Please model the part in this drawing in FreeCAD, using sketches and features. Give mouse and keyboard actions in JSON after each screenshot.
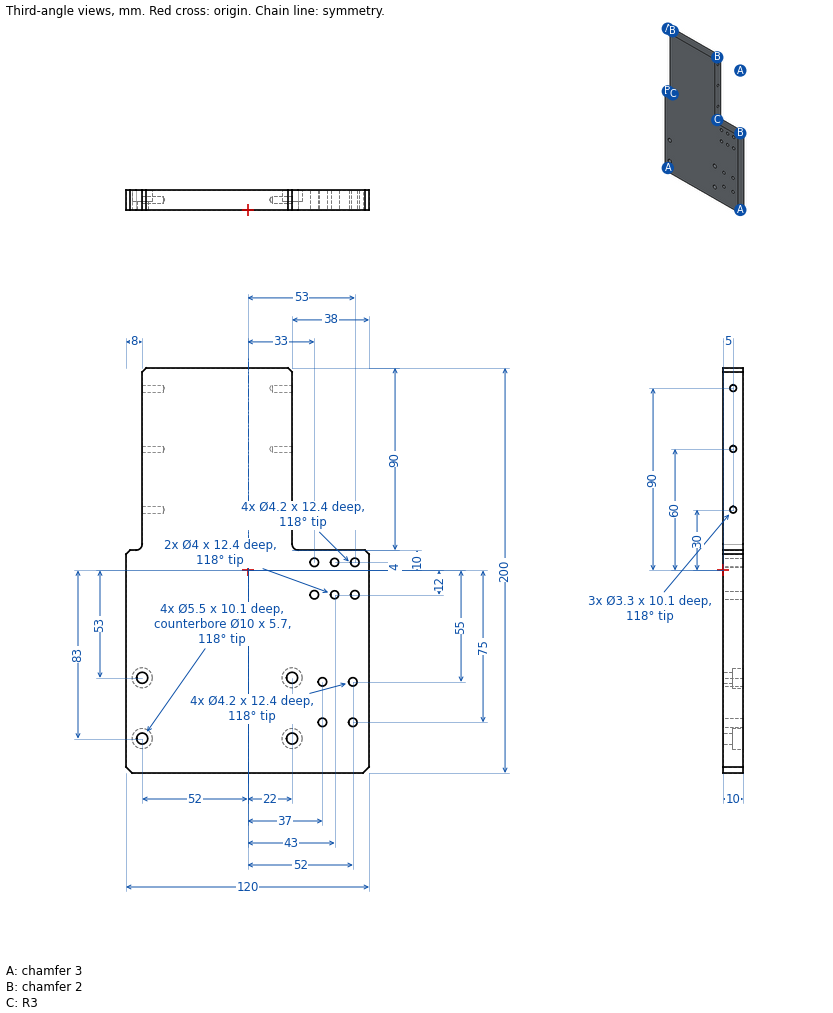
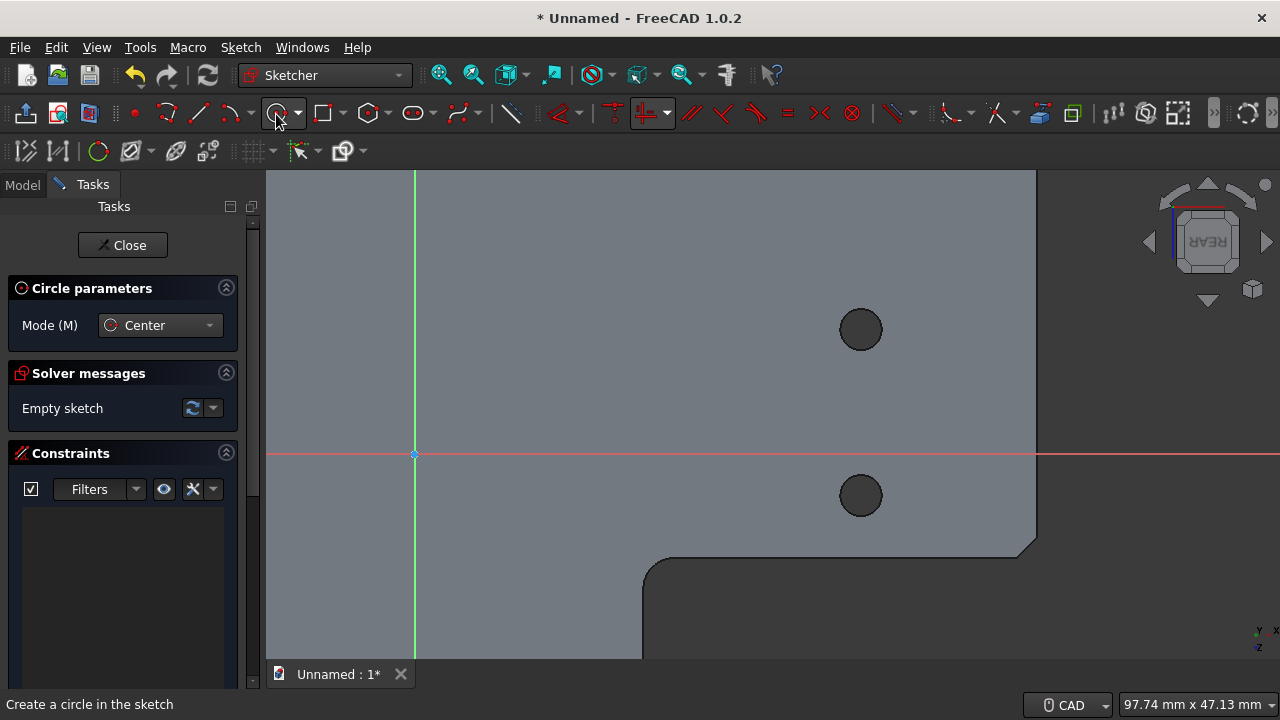
{"action": "left_click", "coordinate": [965, 496]}
{"action": "left_click", "coordinate": [980, 480]}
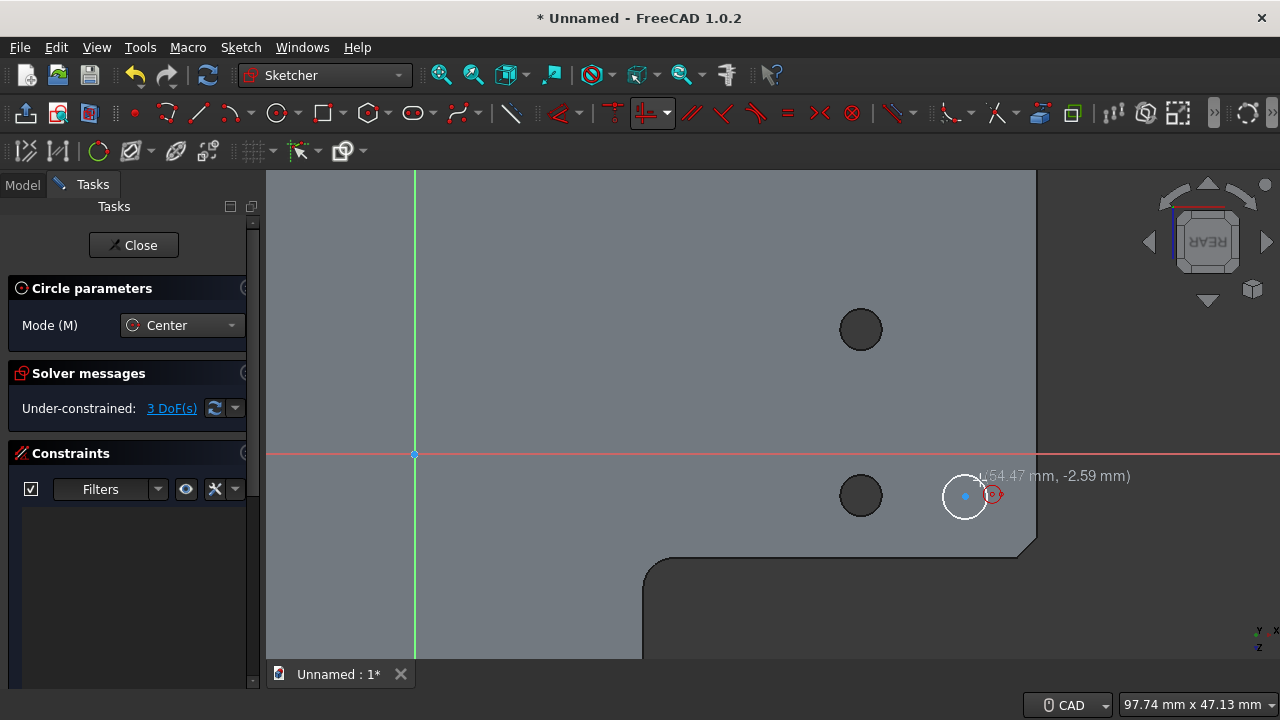
{"action": "left_click", "coordinate": [757, 496]}
{"action": "left_click", "coordinate": [773, 480]}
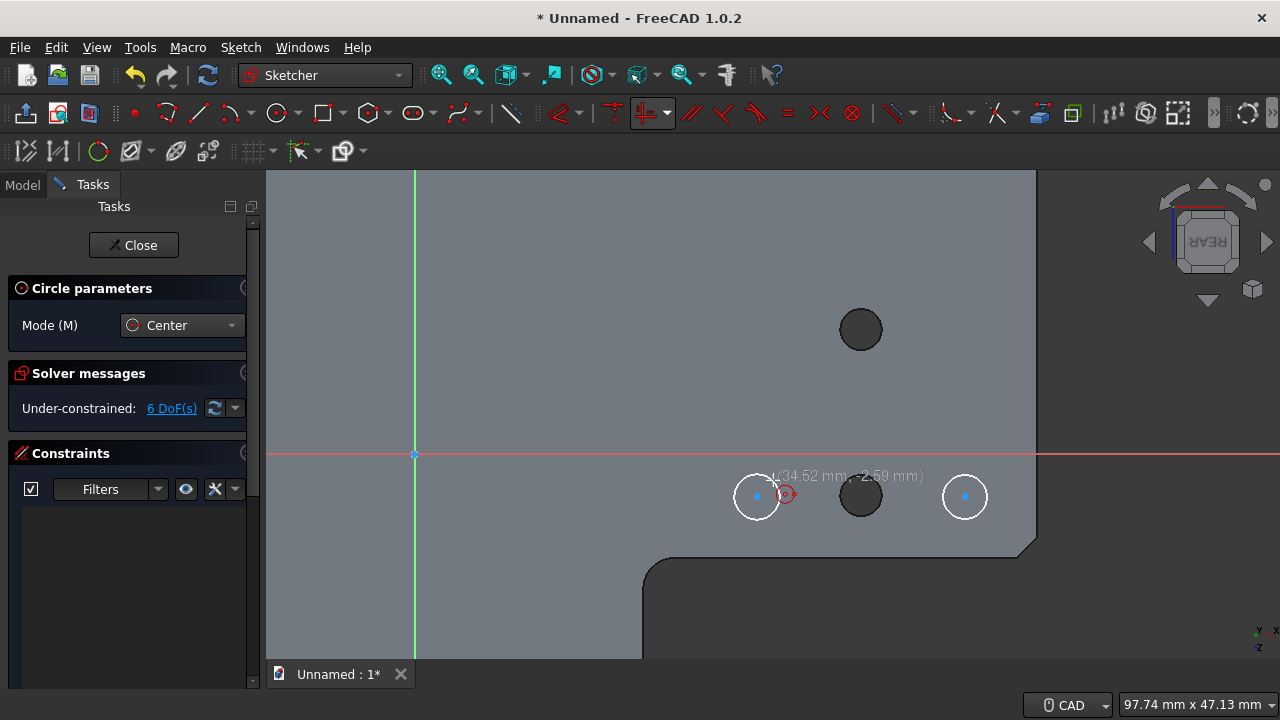
{"action": "left_click", "coordinate": [965, 330]}
{"action": "left_click", "coordinate": [980, 314]}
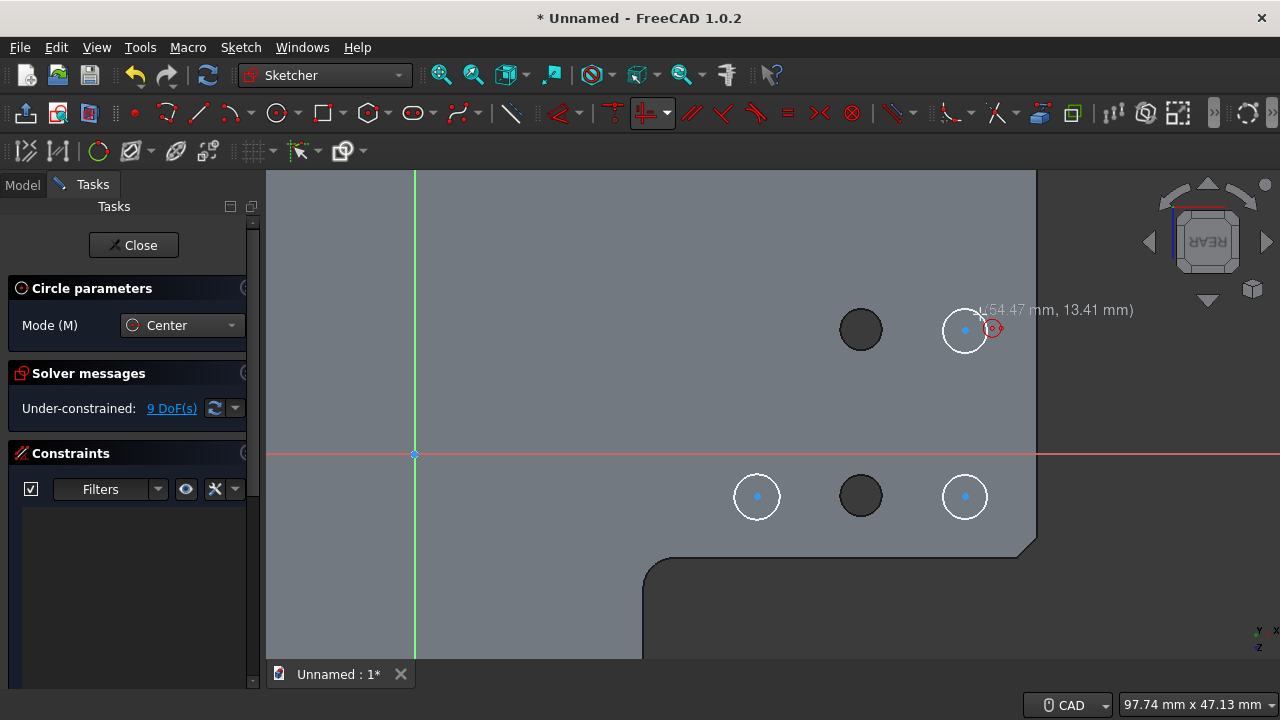
{"action": "left_click", "coordinate": [757, 330]}
{"action": "left_click", "coordinate": [773, 314]}
{"action": "key", "text": "Escape"}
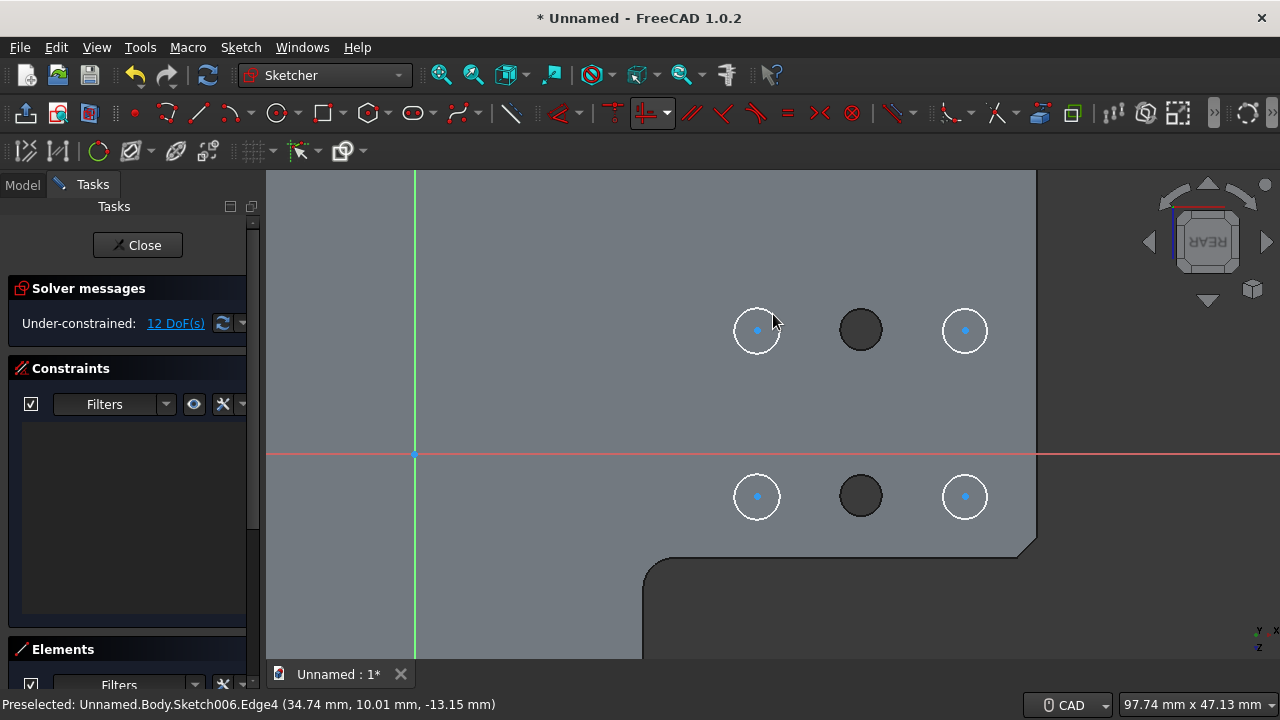
{"action": "left_click", "coordinate": [980, 481]}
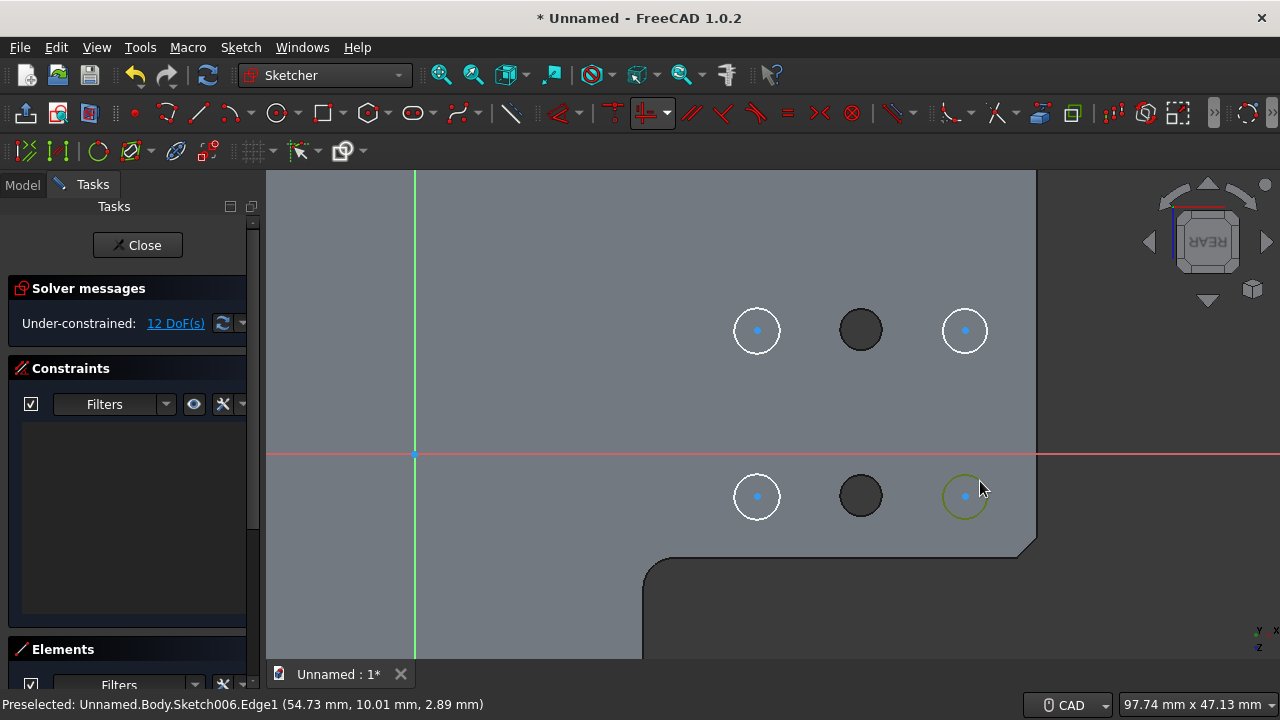
{"action": "left_click", "coordinate": [773, 481]}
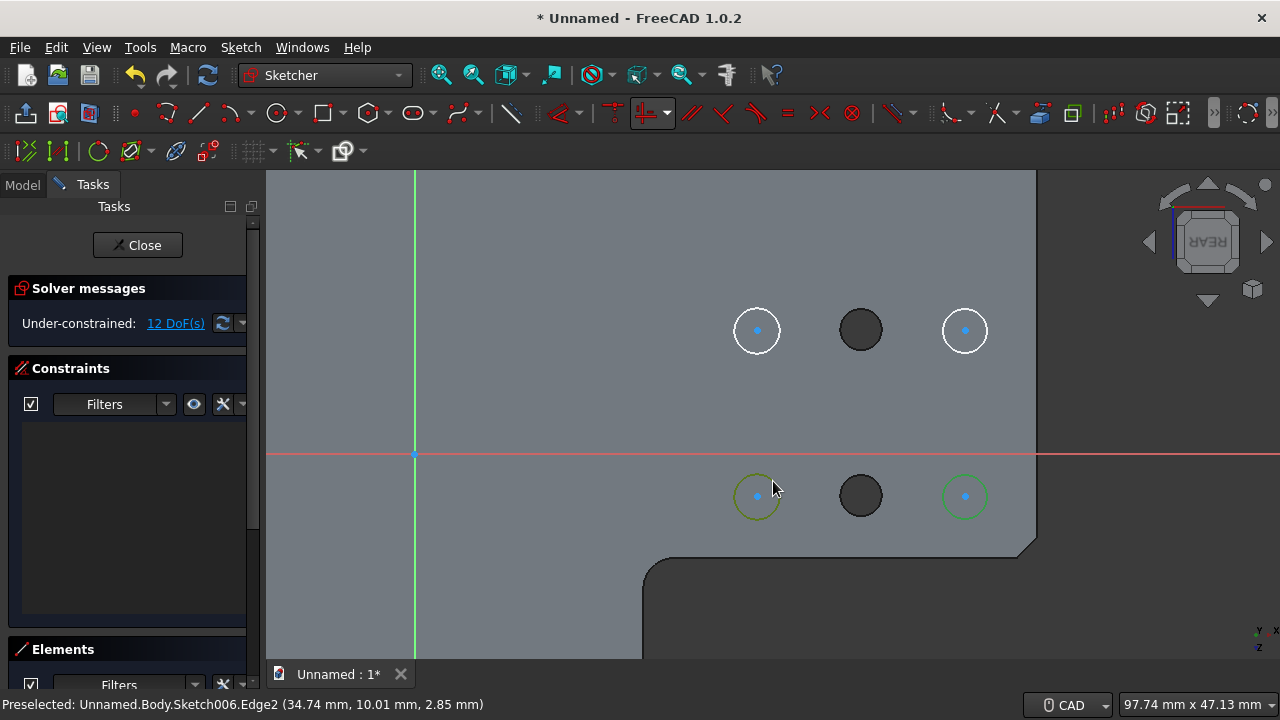
{"action": "left_click", "coordinate": [980, 315]}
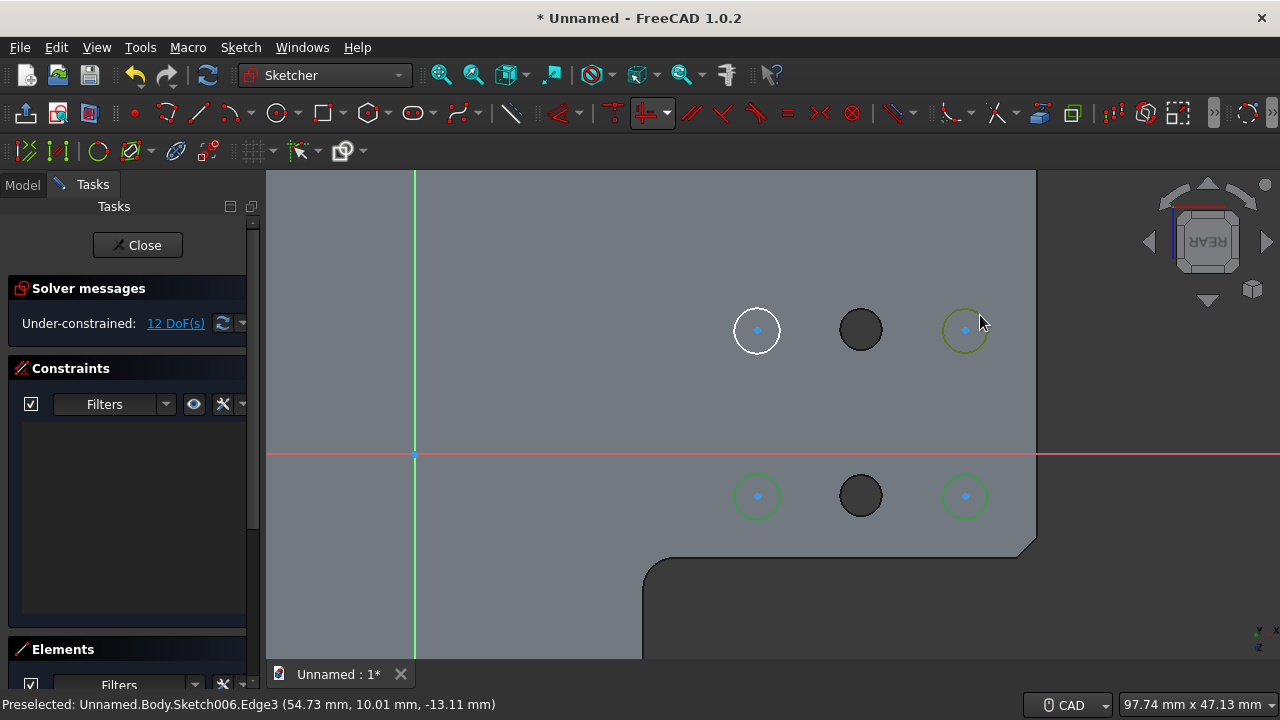
{"action": "left_click", "coordinate": [773, 315]}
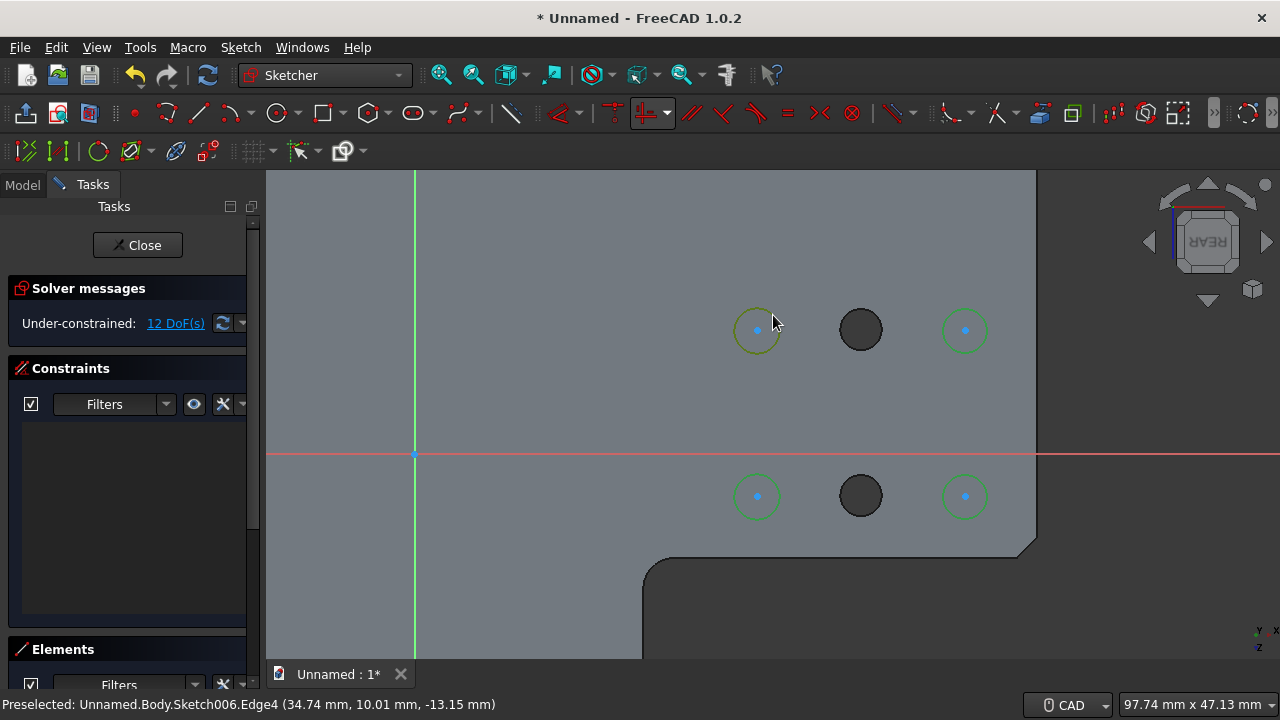
{"action": "key", "text": "e"}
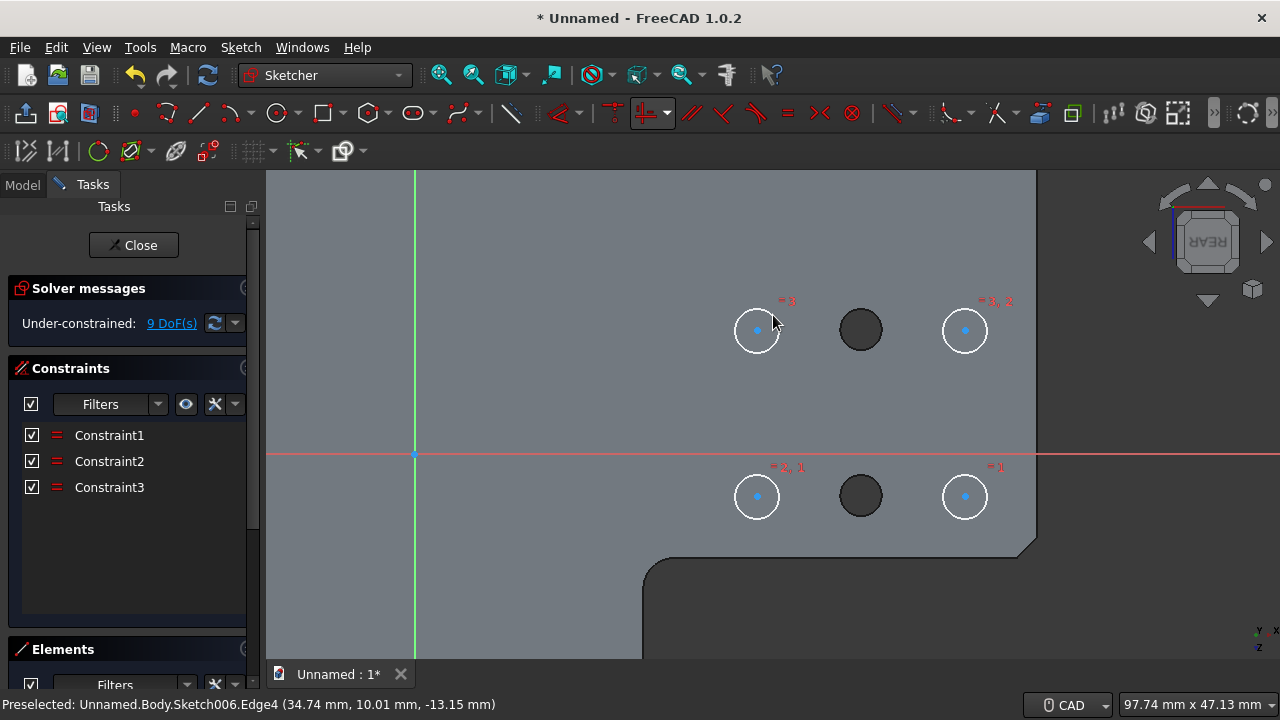
{"action": "left_click", "coordinate": [965, 497]}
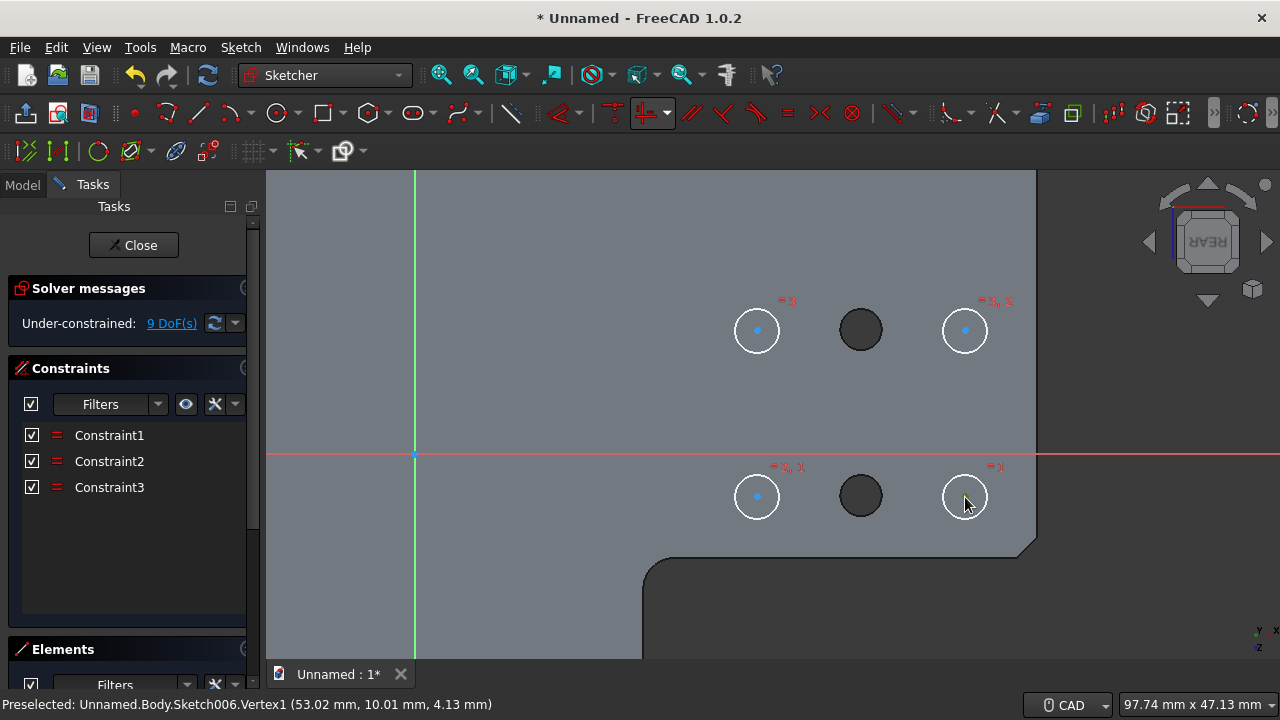
{"action": "left_click", "coordinate": [757, 497]}